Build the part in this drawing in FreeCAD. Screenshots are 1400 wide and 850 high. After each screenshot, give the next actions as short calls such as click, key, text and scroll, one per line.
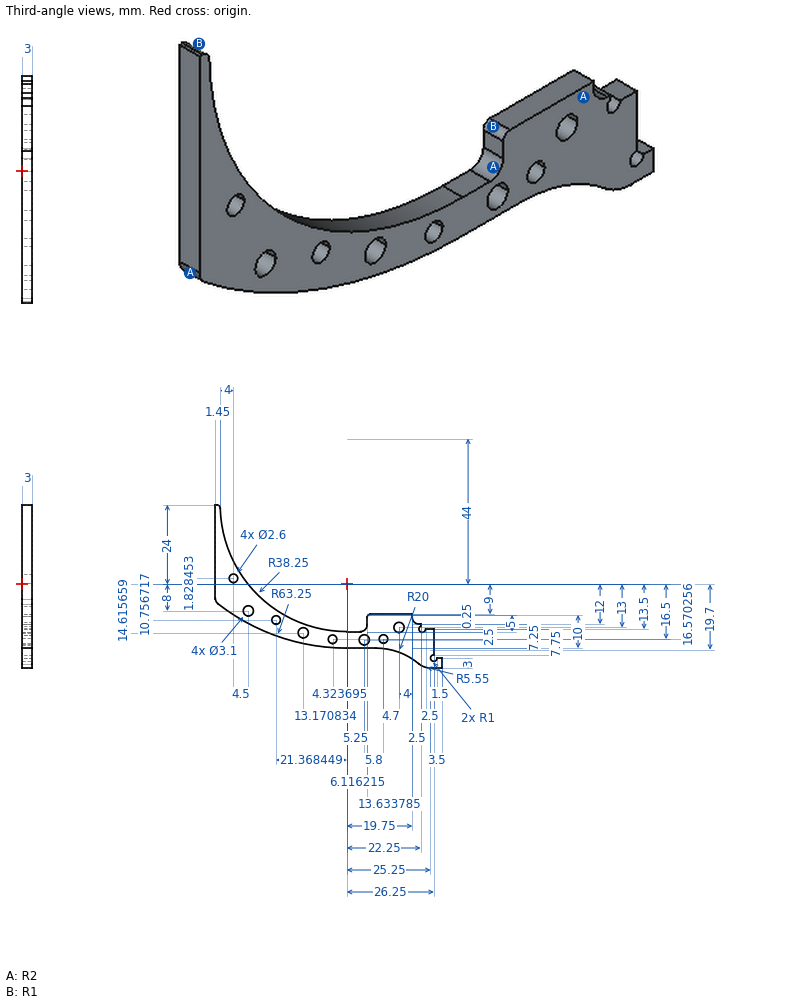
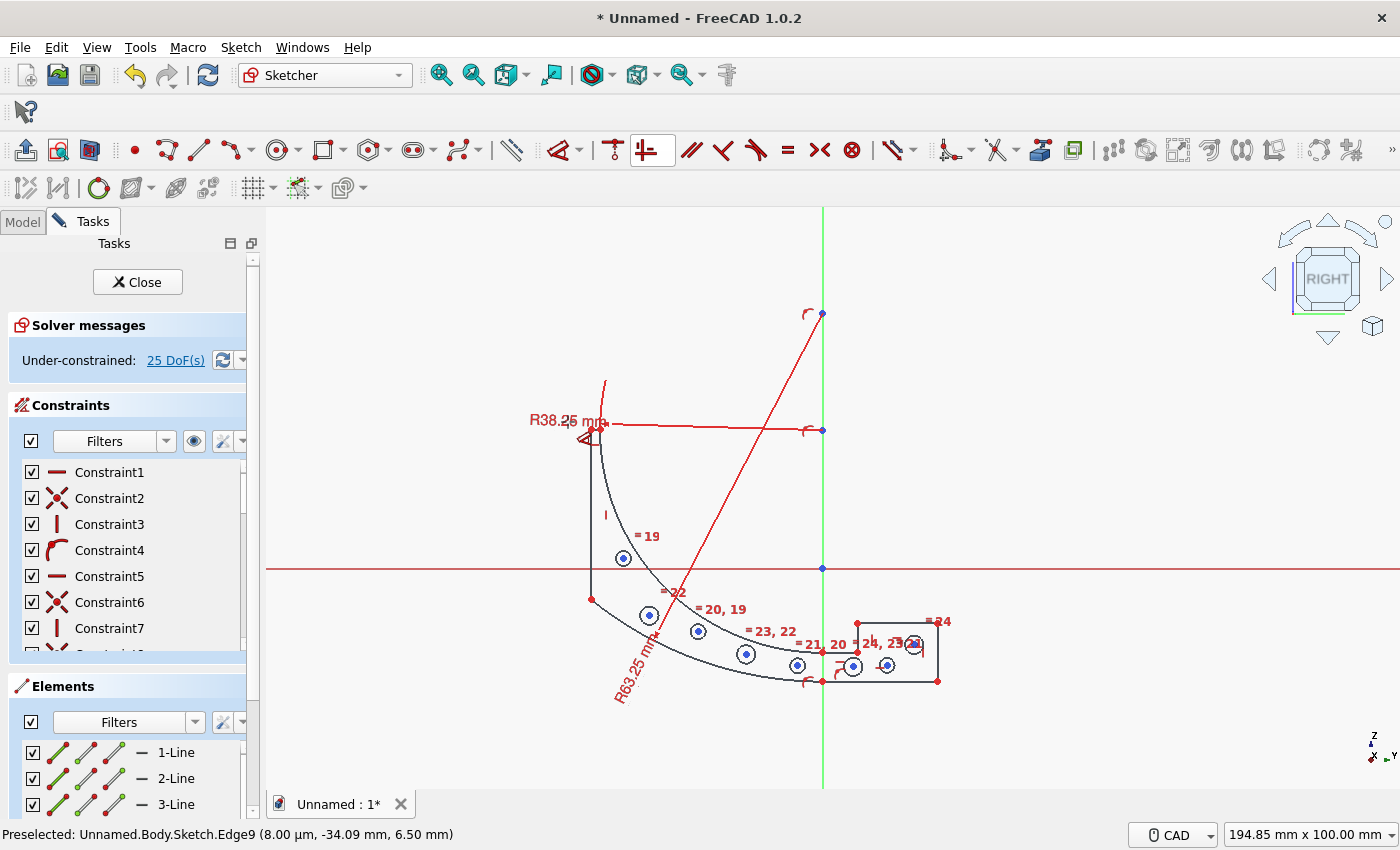
scroll(624, 551, up, 5)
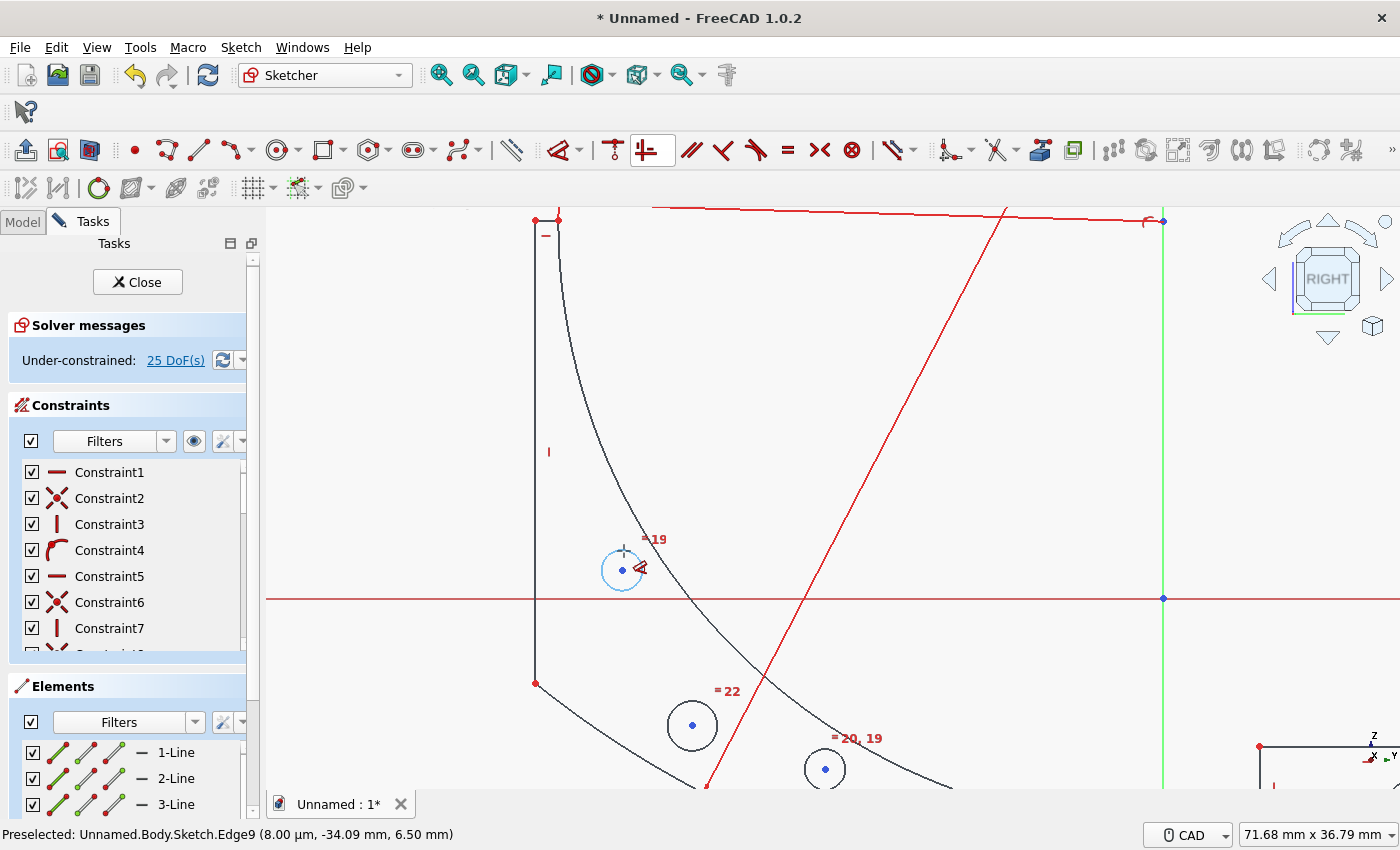
click(623, 550)
click(599, 523)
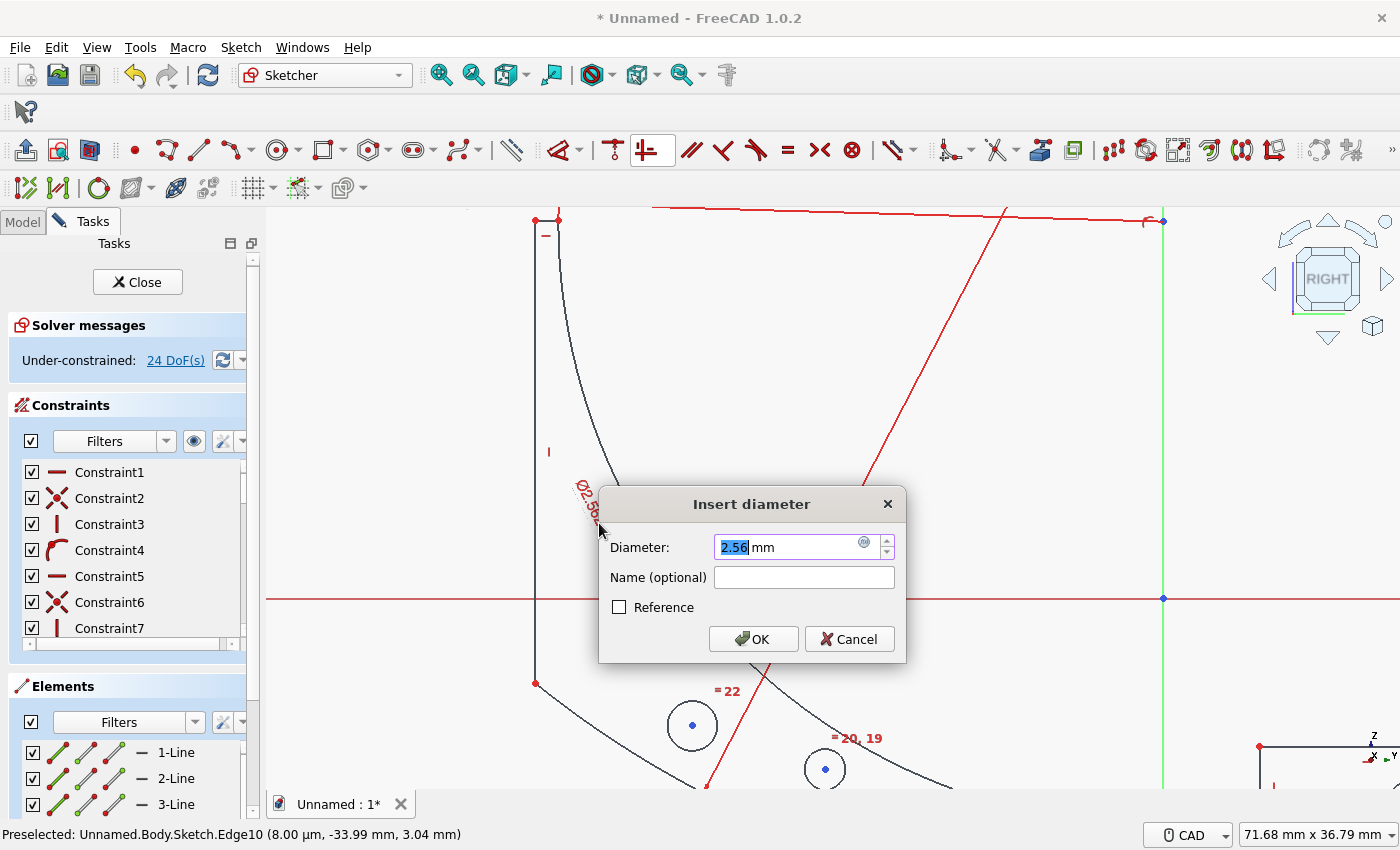
text(2.6)
key(Return)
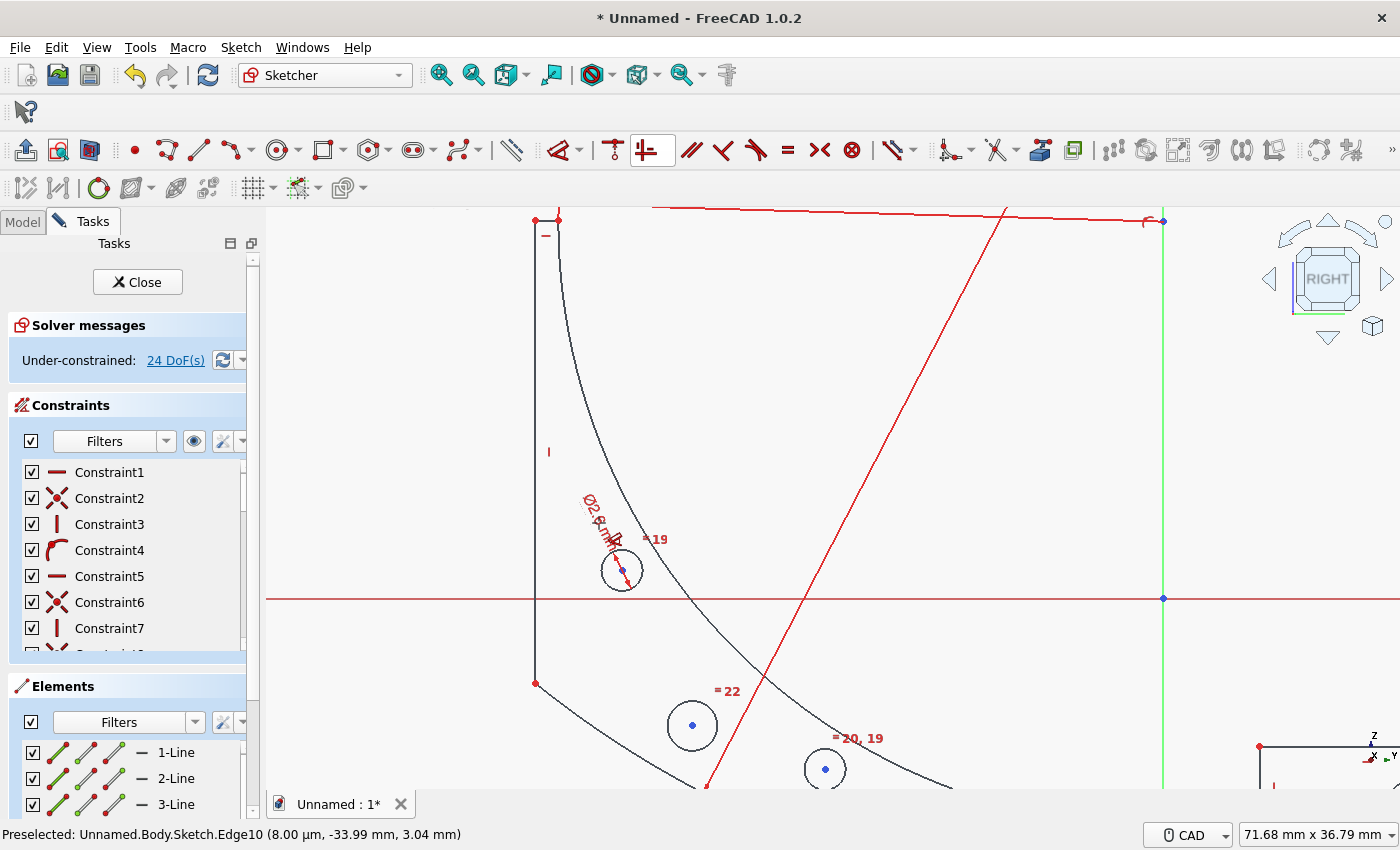
click(710, 708)
click(732, 685)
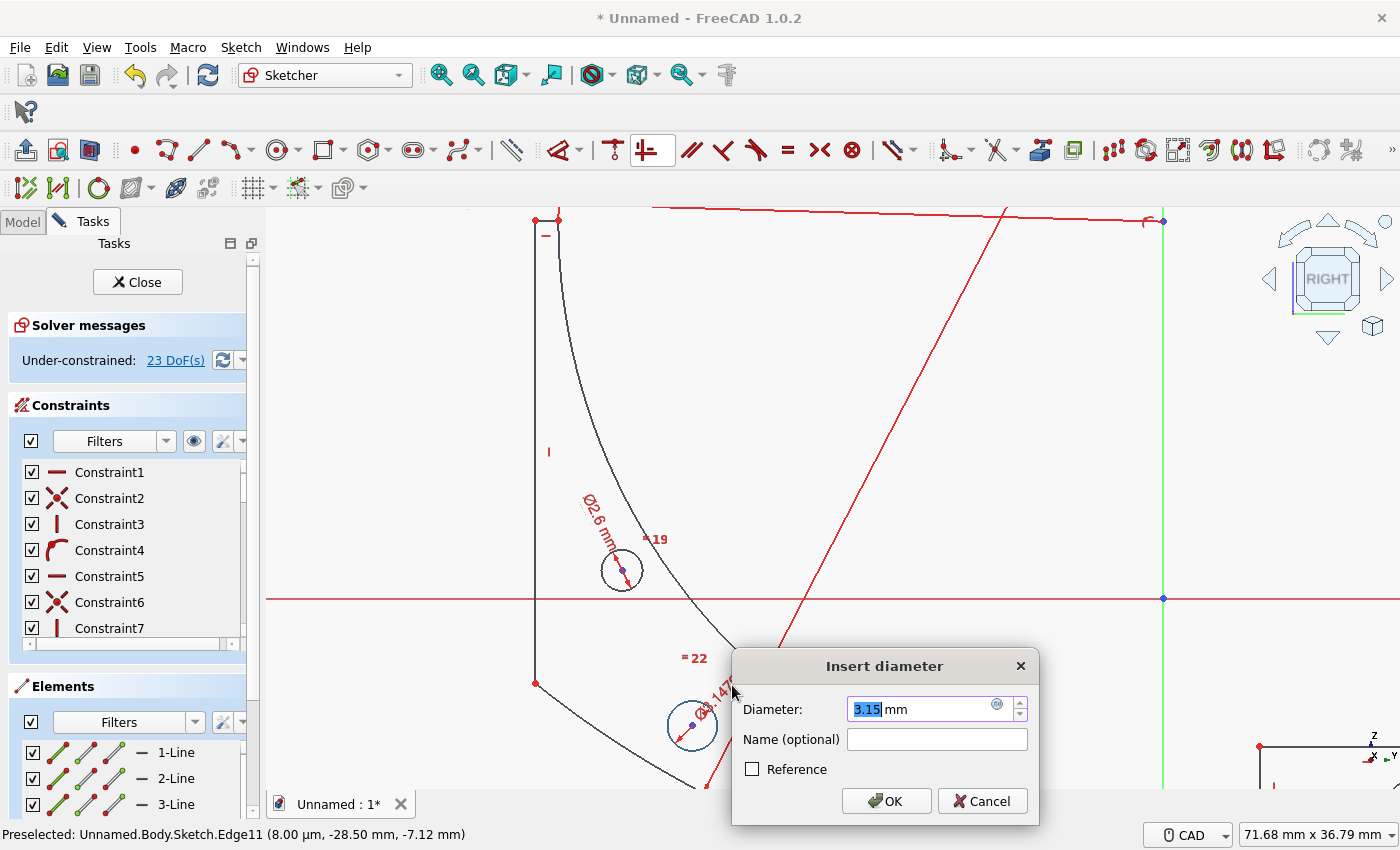
text(3.1)
key(Return)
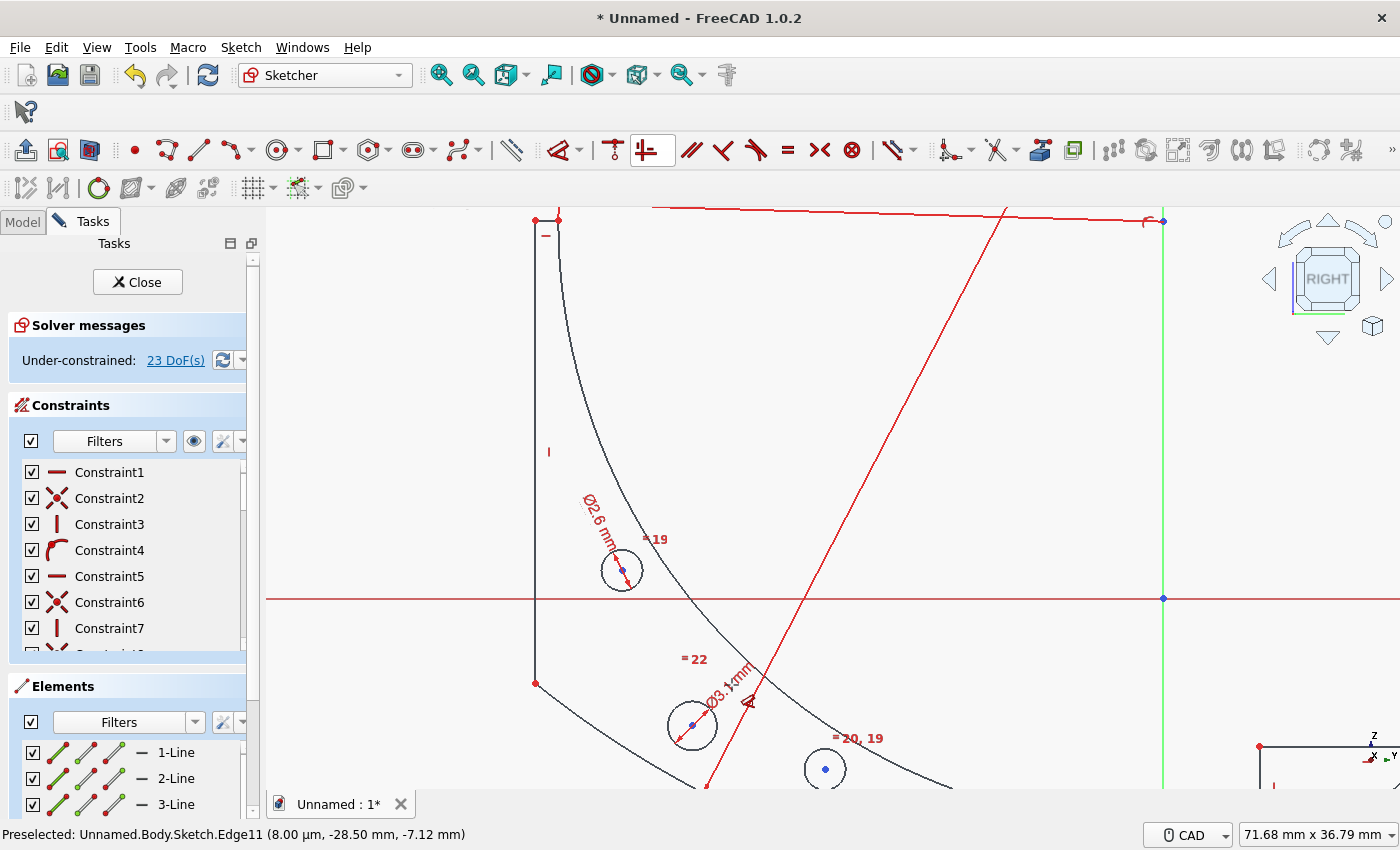
scroll(471, 421, down, 3)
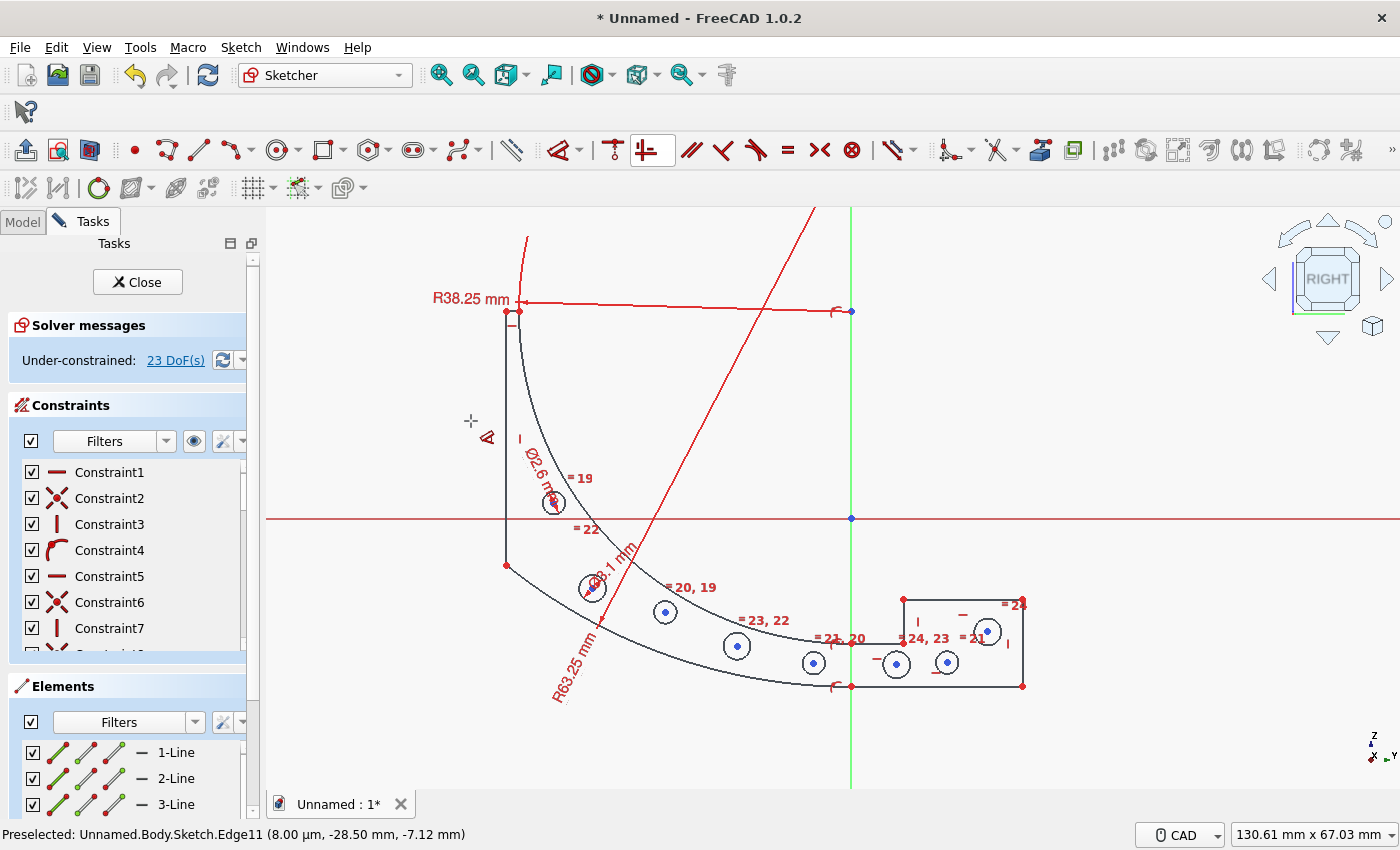
click(904, 613)
click(938, 622)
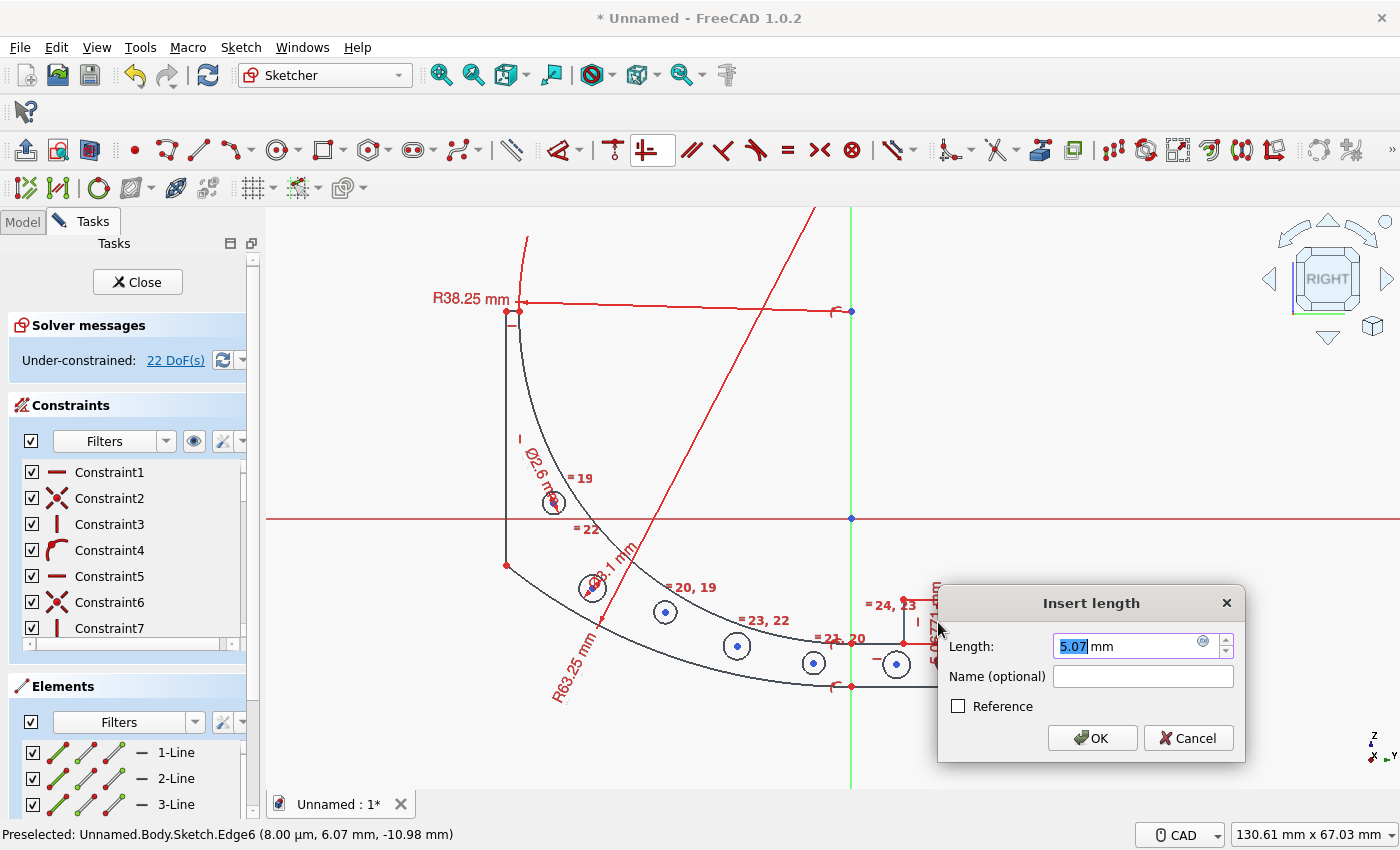
text(5)
key(Return)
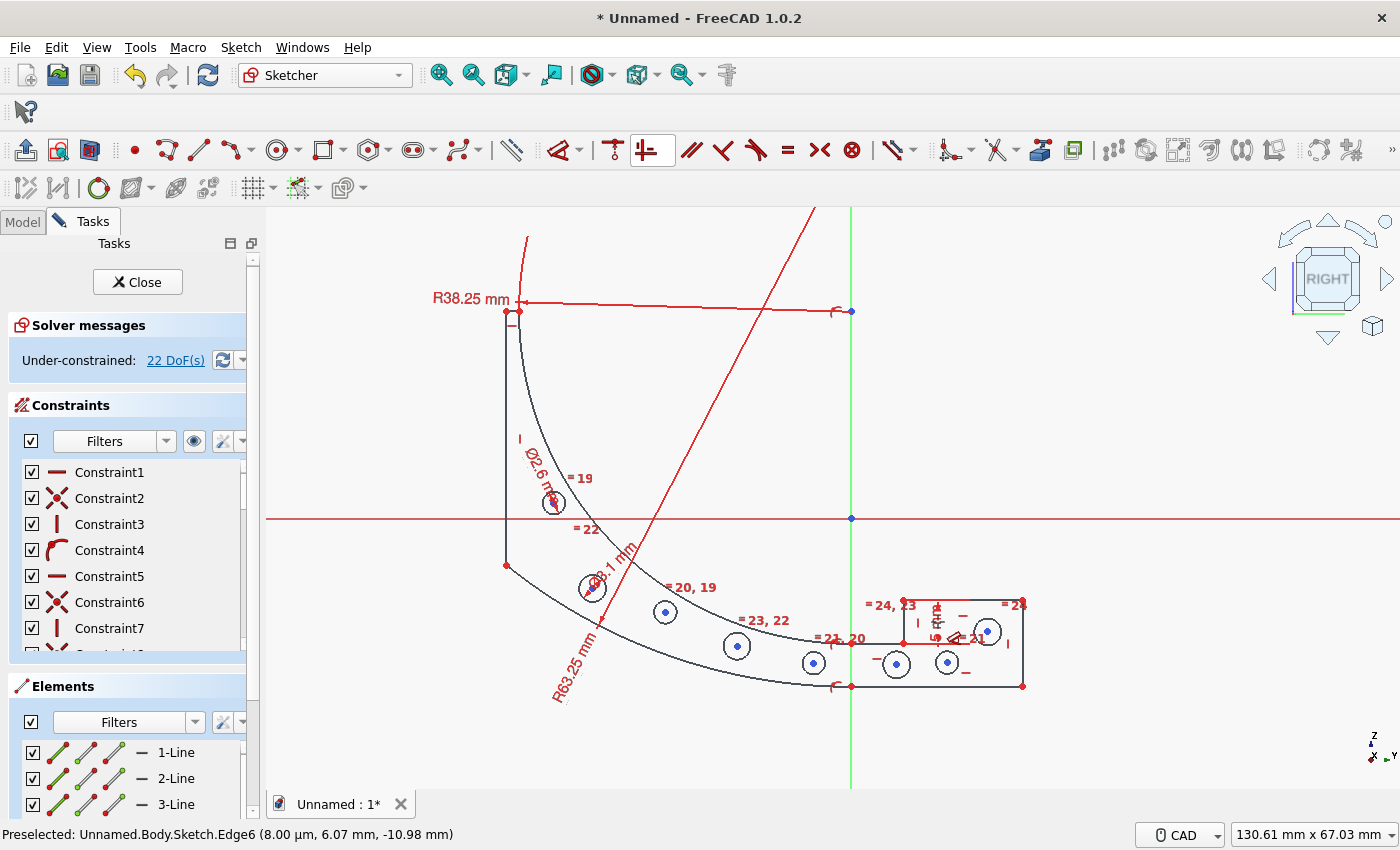
click(593, 589)
click(559, 538)